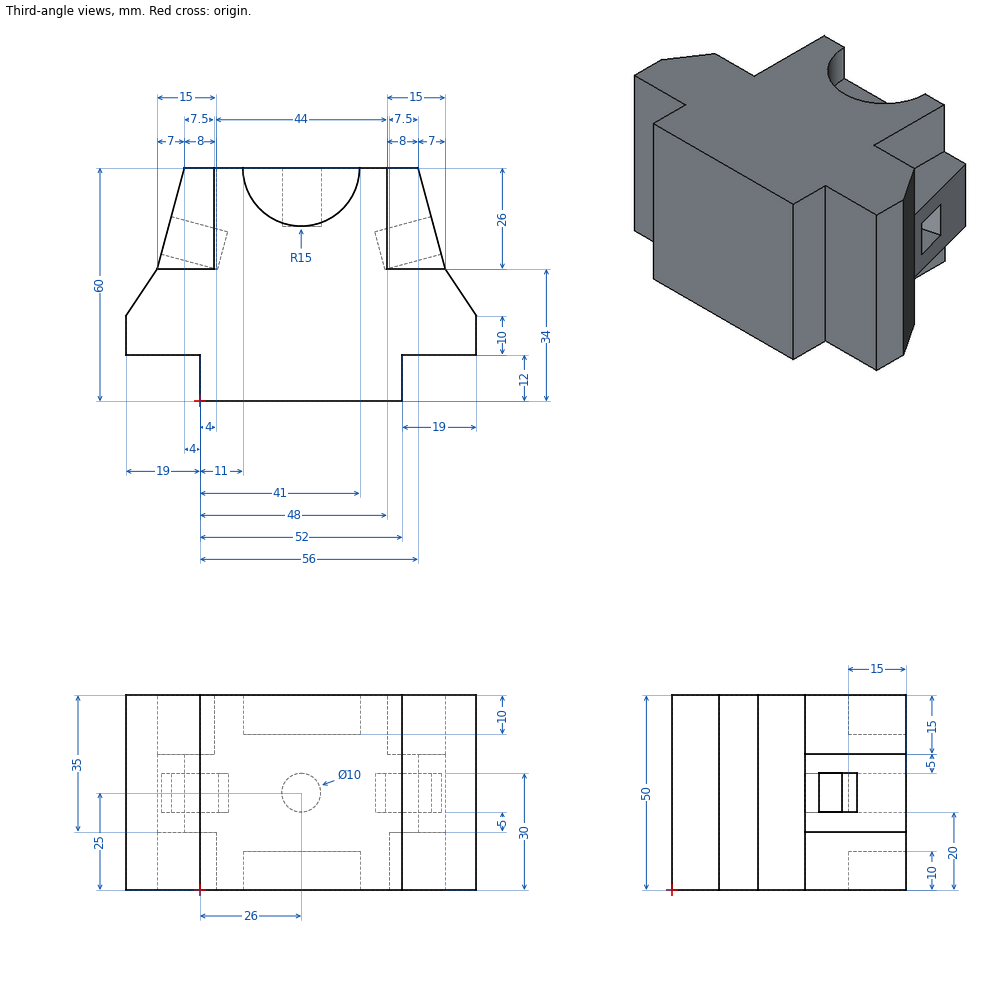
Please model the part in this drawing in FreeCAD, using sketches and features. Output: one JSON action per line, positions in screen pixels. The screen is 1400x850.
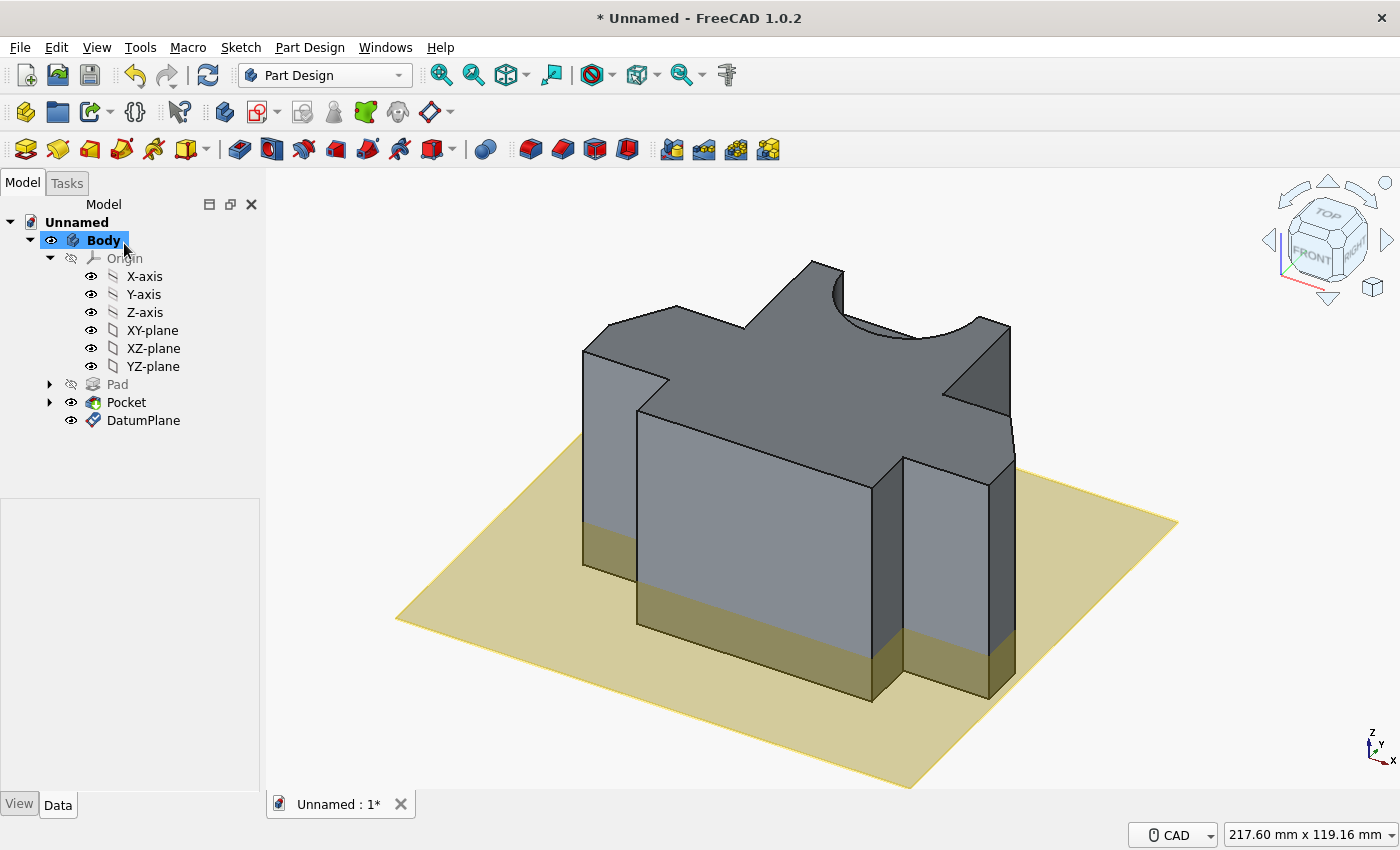
{"action": "left_click", "coordinate": [116, 420]}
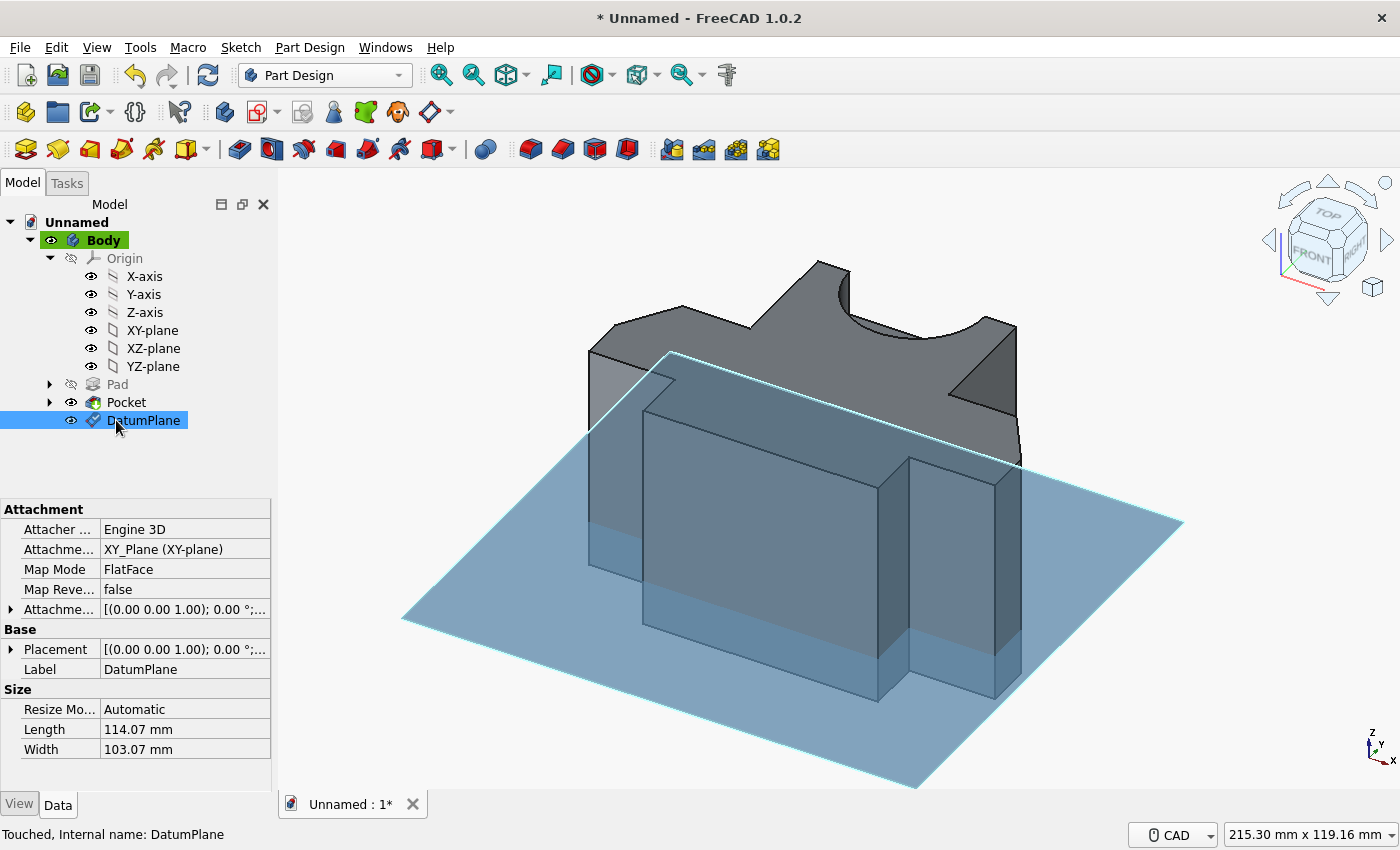
{"action": "left_click", "coordinate": [258, 112]}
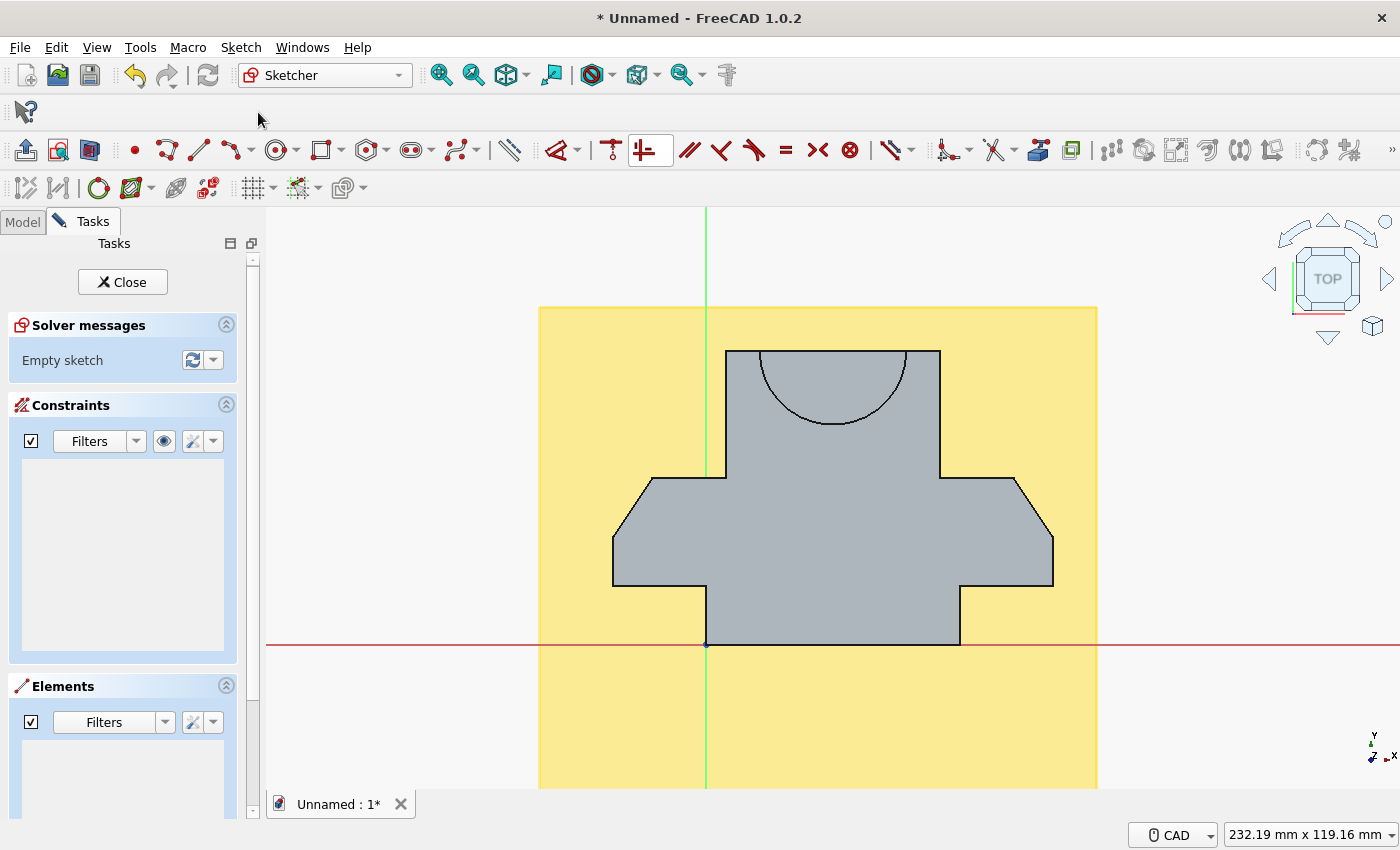
{"action": "left_click", "coordinate": [90, 150]}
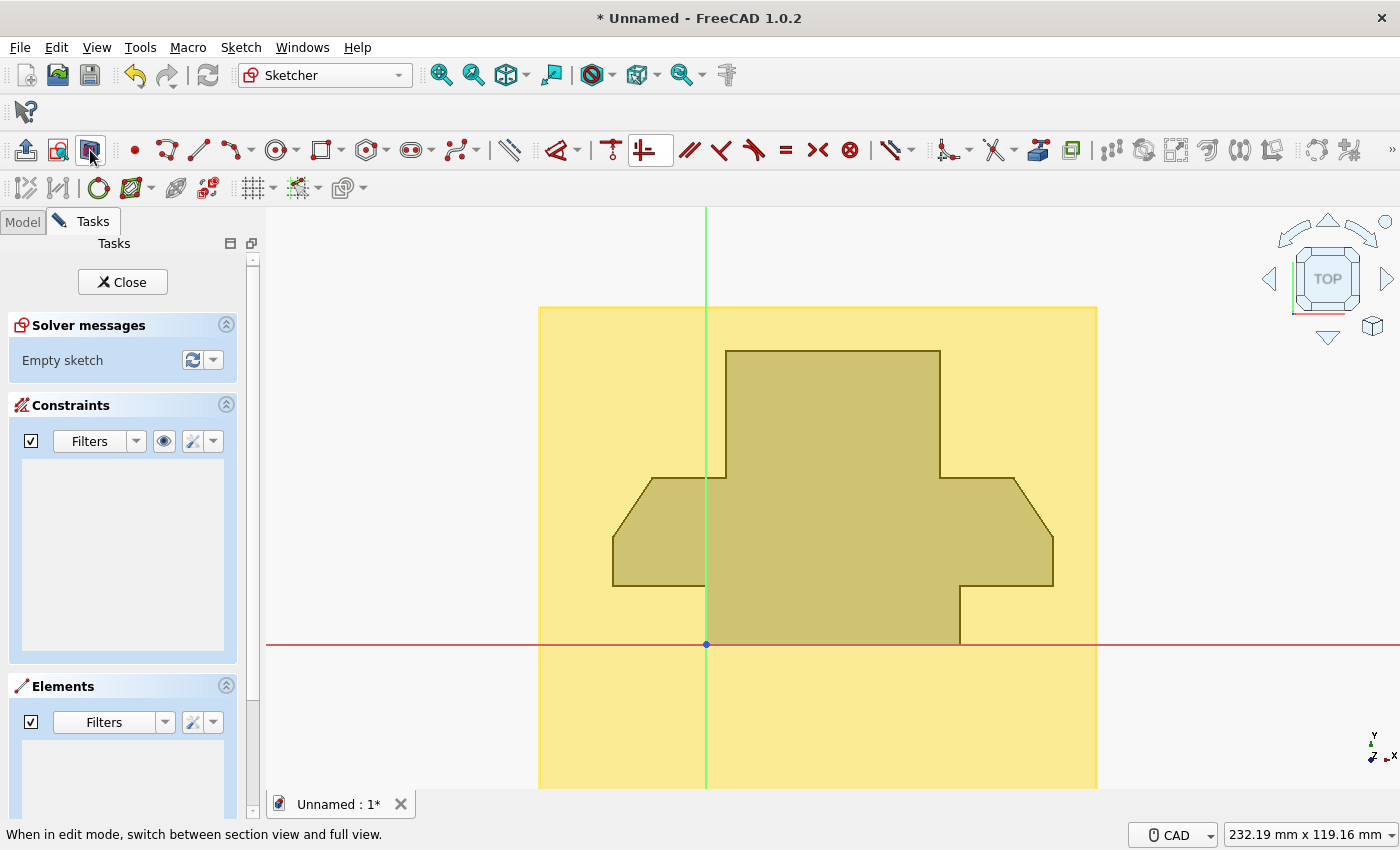
{"action": "left_click", "coordinate": [200, 150]}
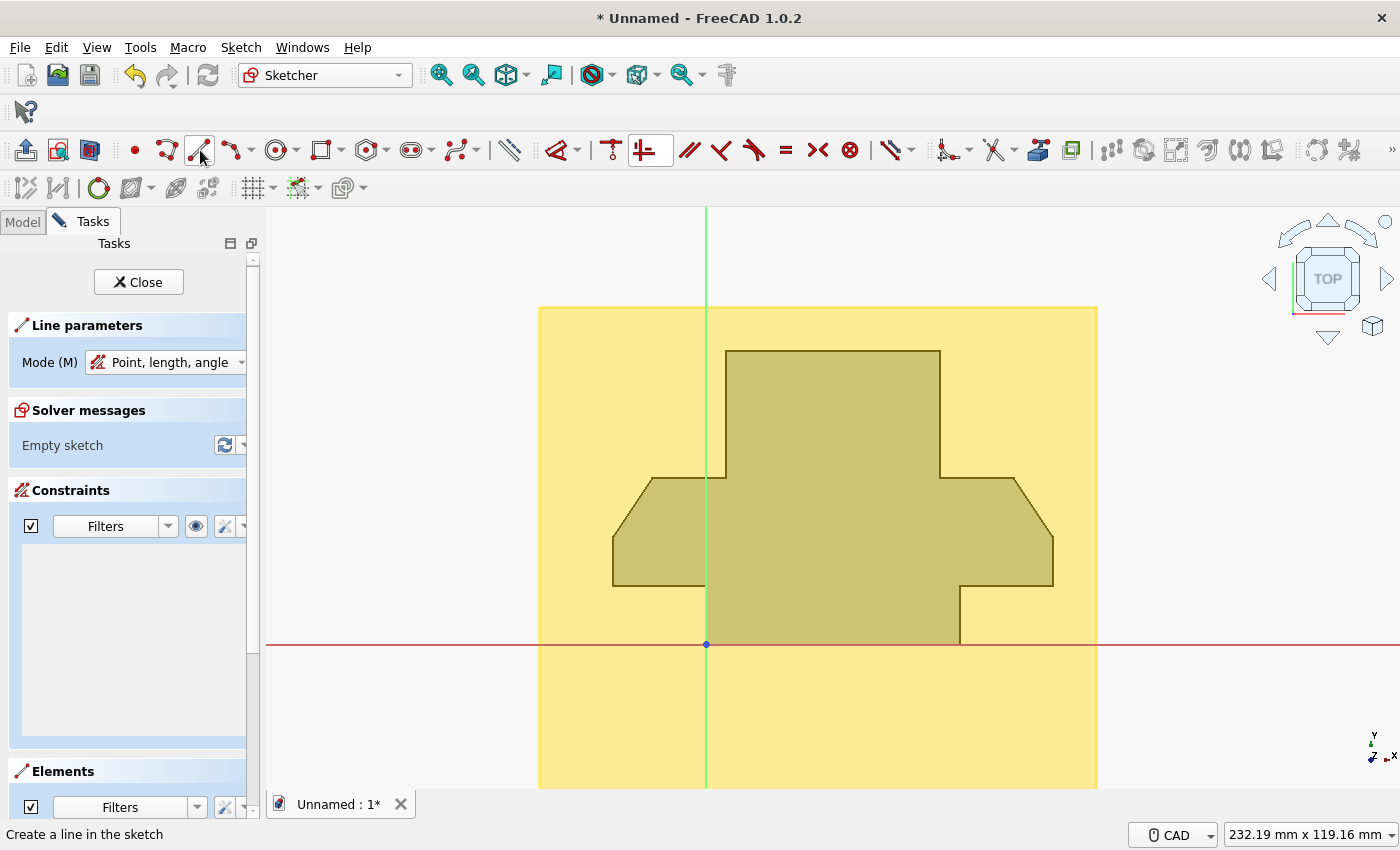
{"action": "left_click", "coordinate": [760, 351]}
{"action": "left_click", "coordinate": [906, 351]}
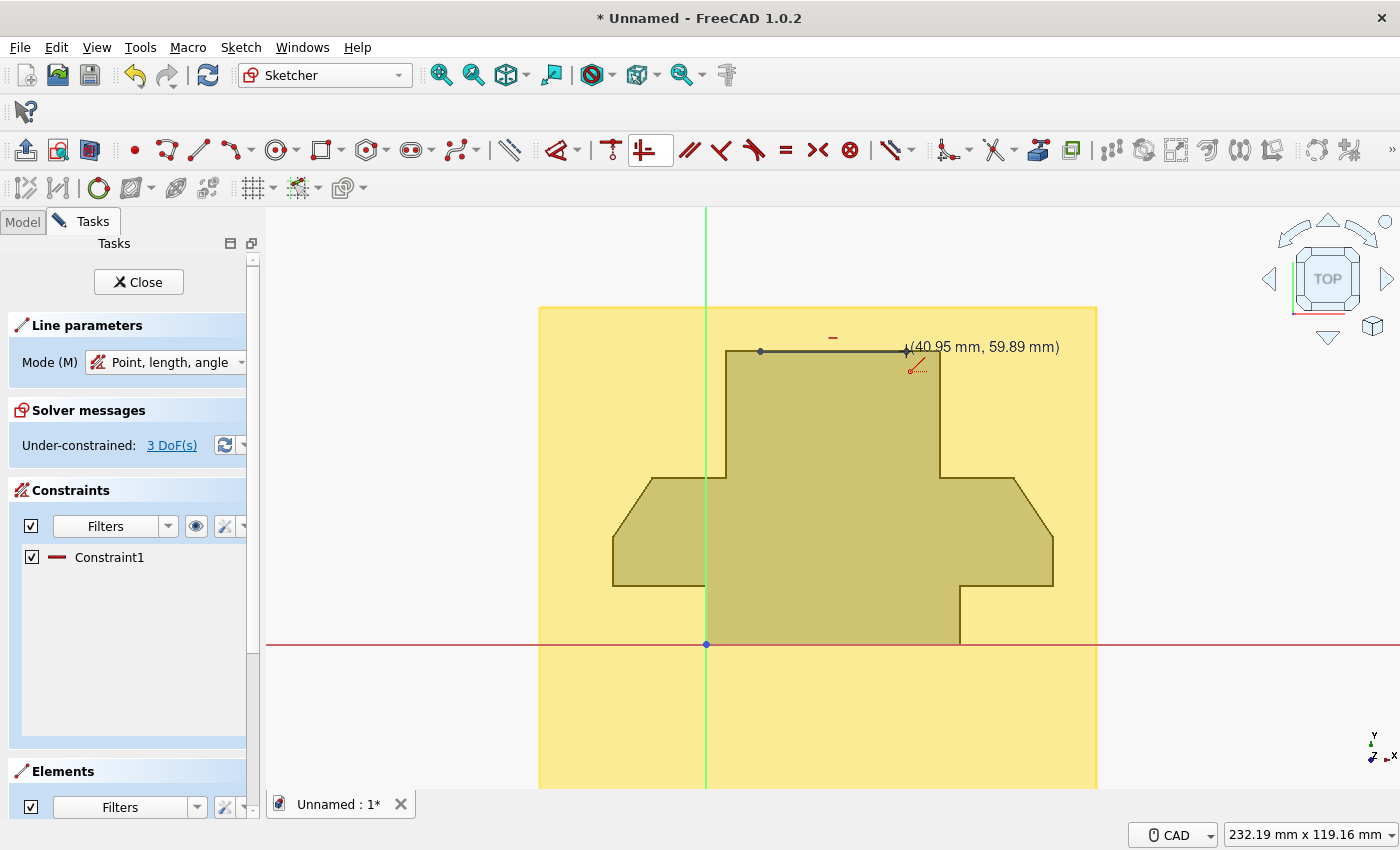
{"action": "left_click", "coordinate": [232, 150]}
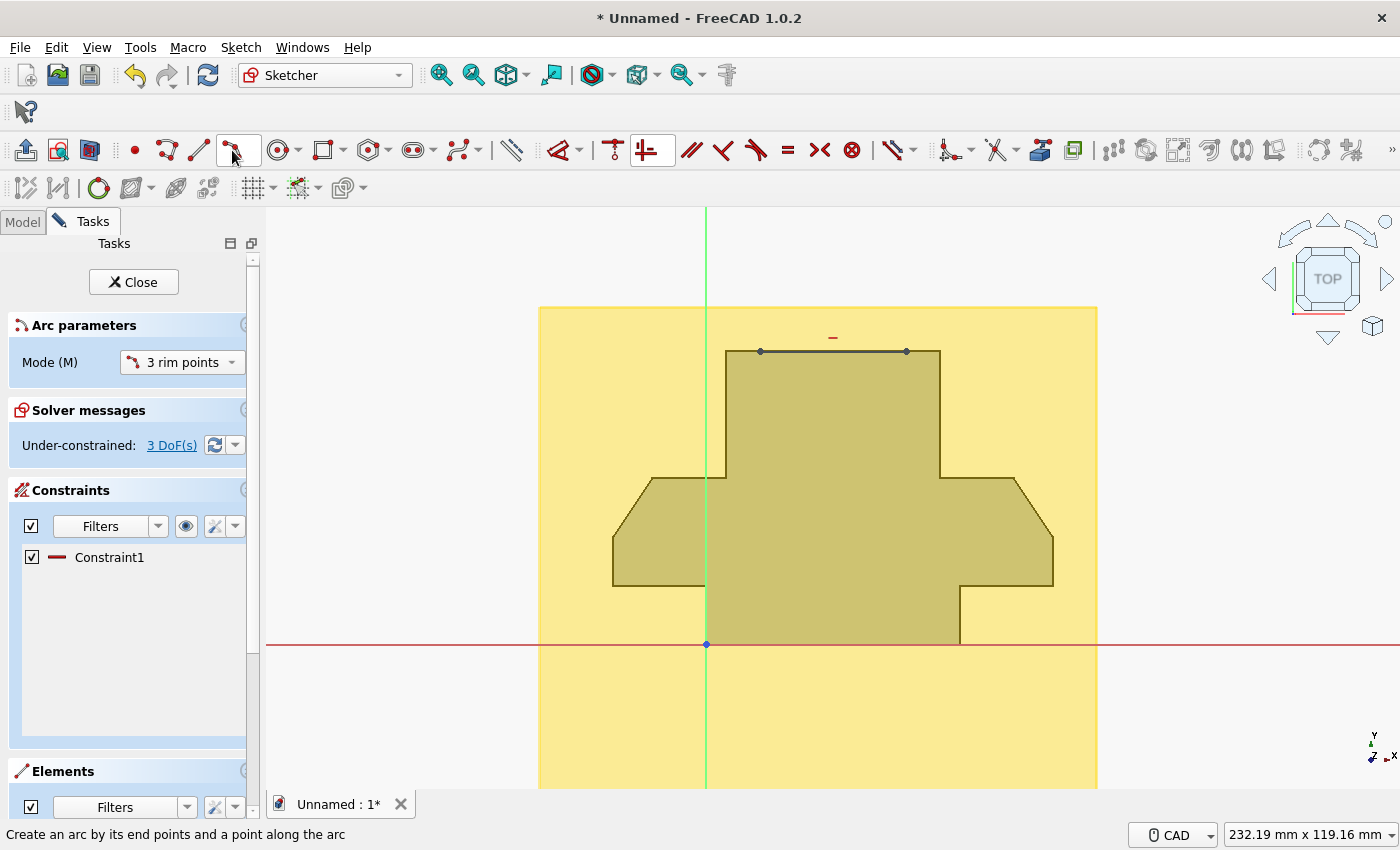
{"action": "left_click", "coordinate": [906, 352]}
{"action": "left_click", "coordinate": [760, 352]}
{"action": "left_click", "coordinate": [833, 425]}
{"action": "key", "text": "Escape"}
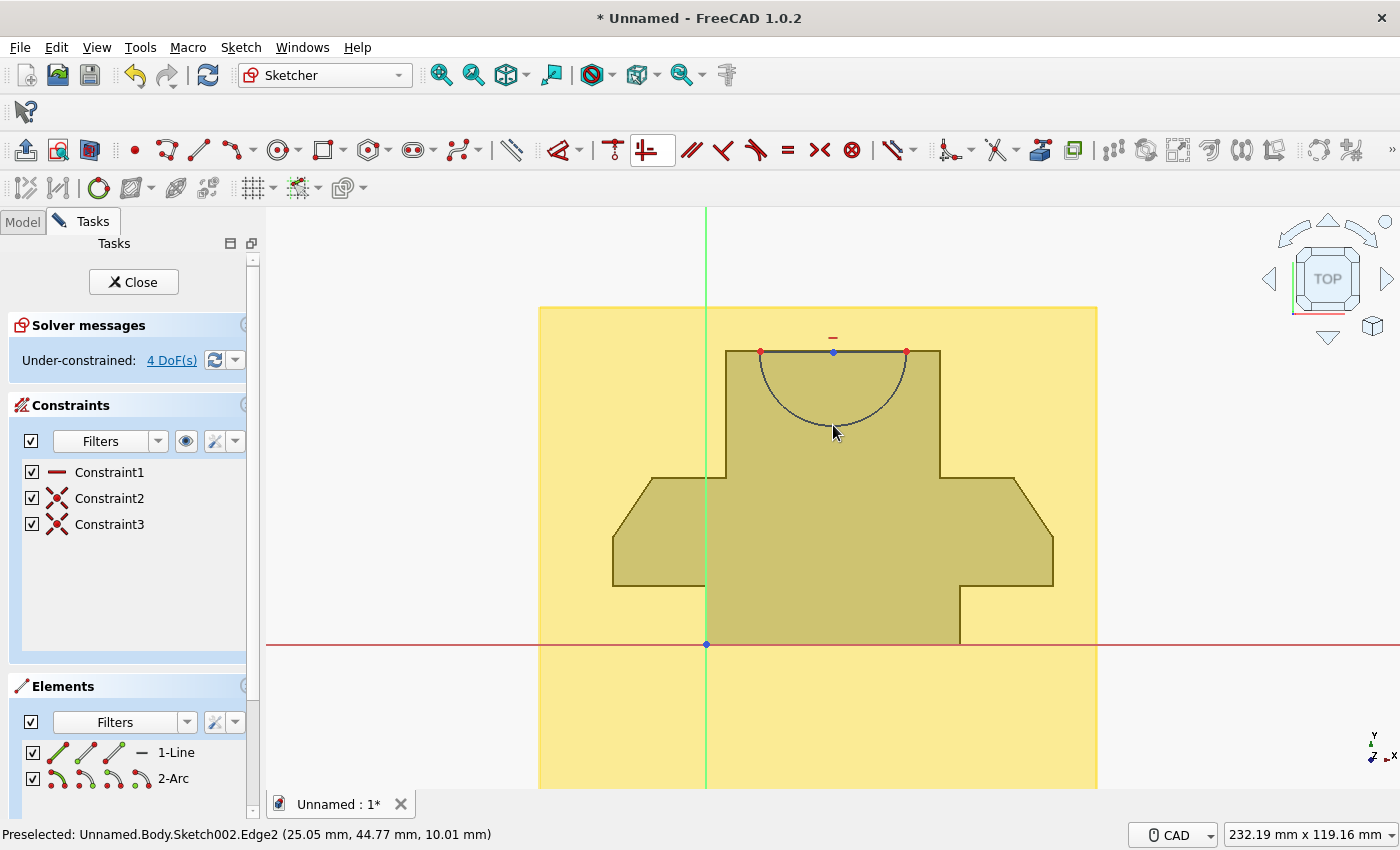
{"action": "left_click", "coordinate": [558, 150]}